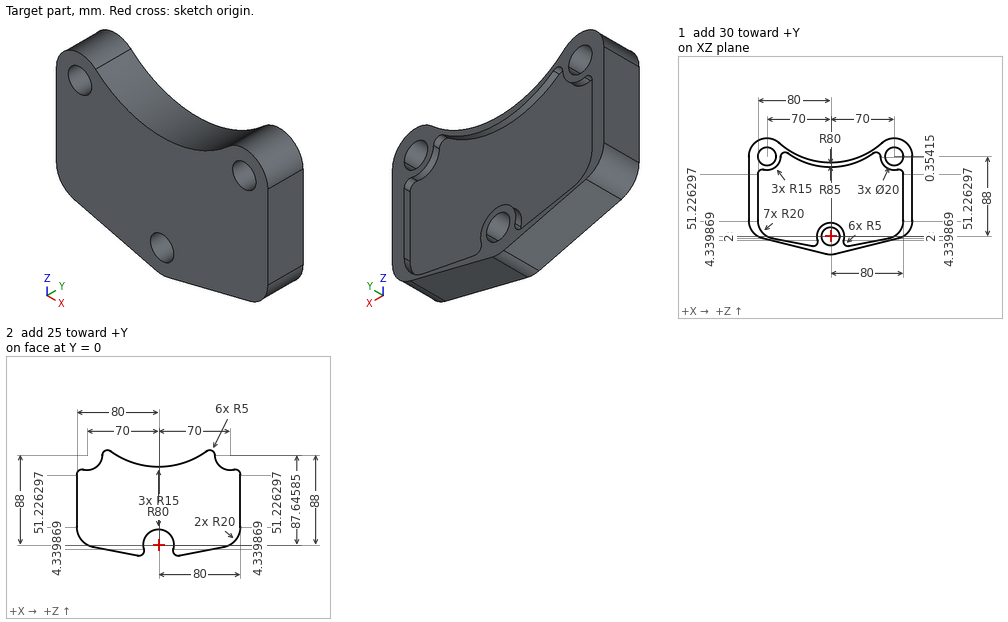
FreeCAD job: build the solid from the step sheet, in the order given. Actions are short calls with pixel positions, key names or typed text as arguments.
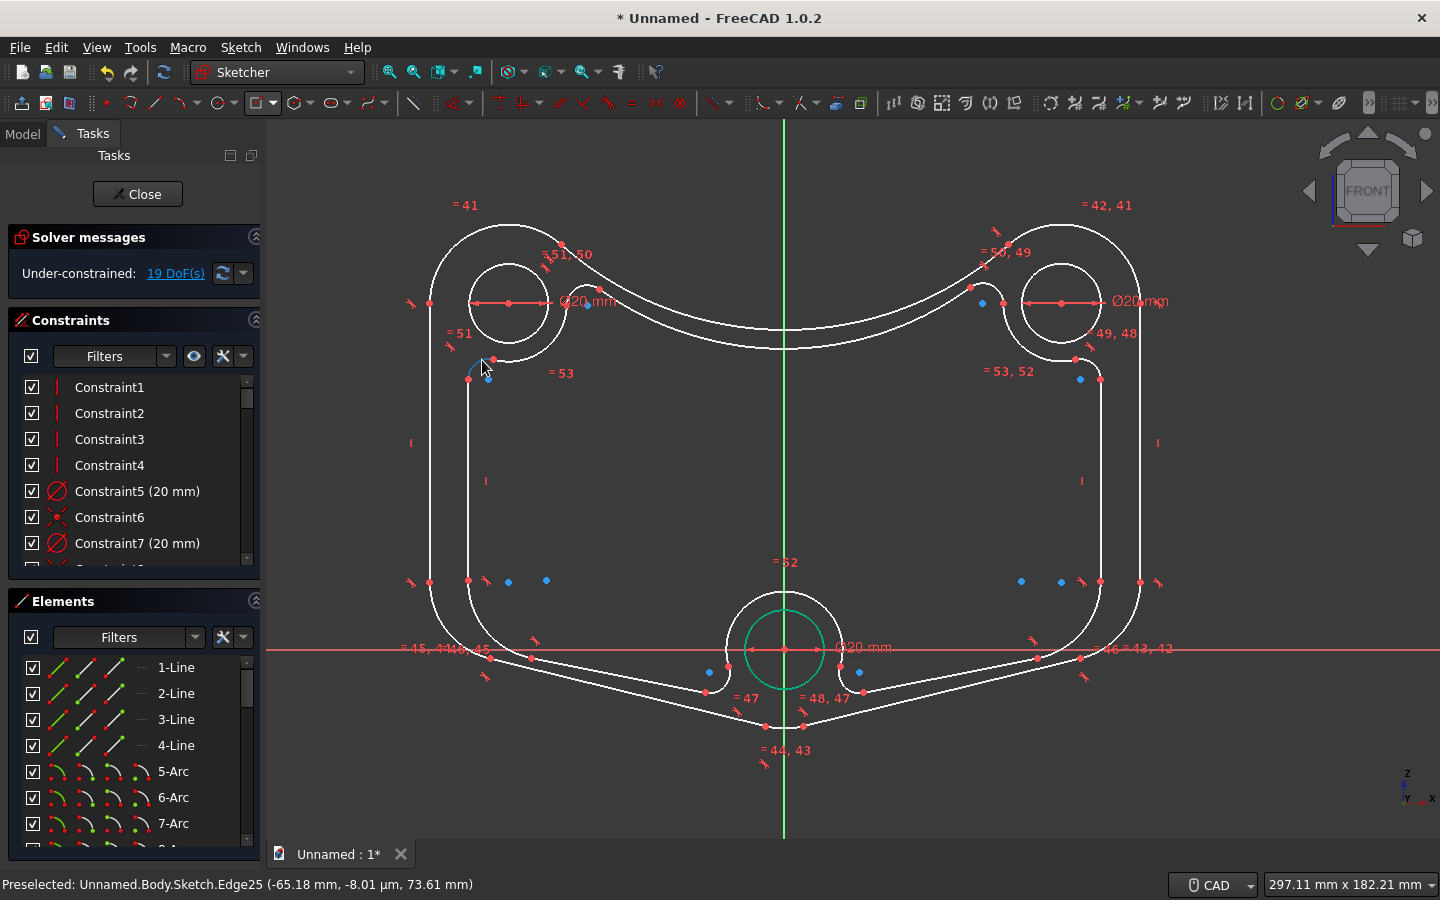
scroll(785, 719, down, 2)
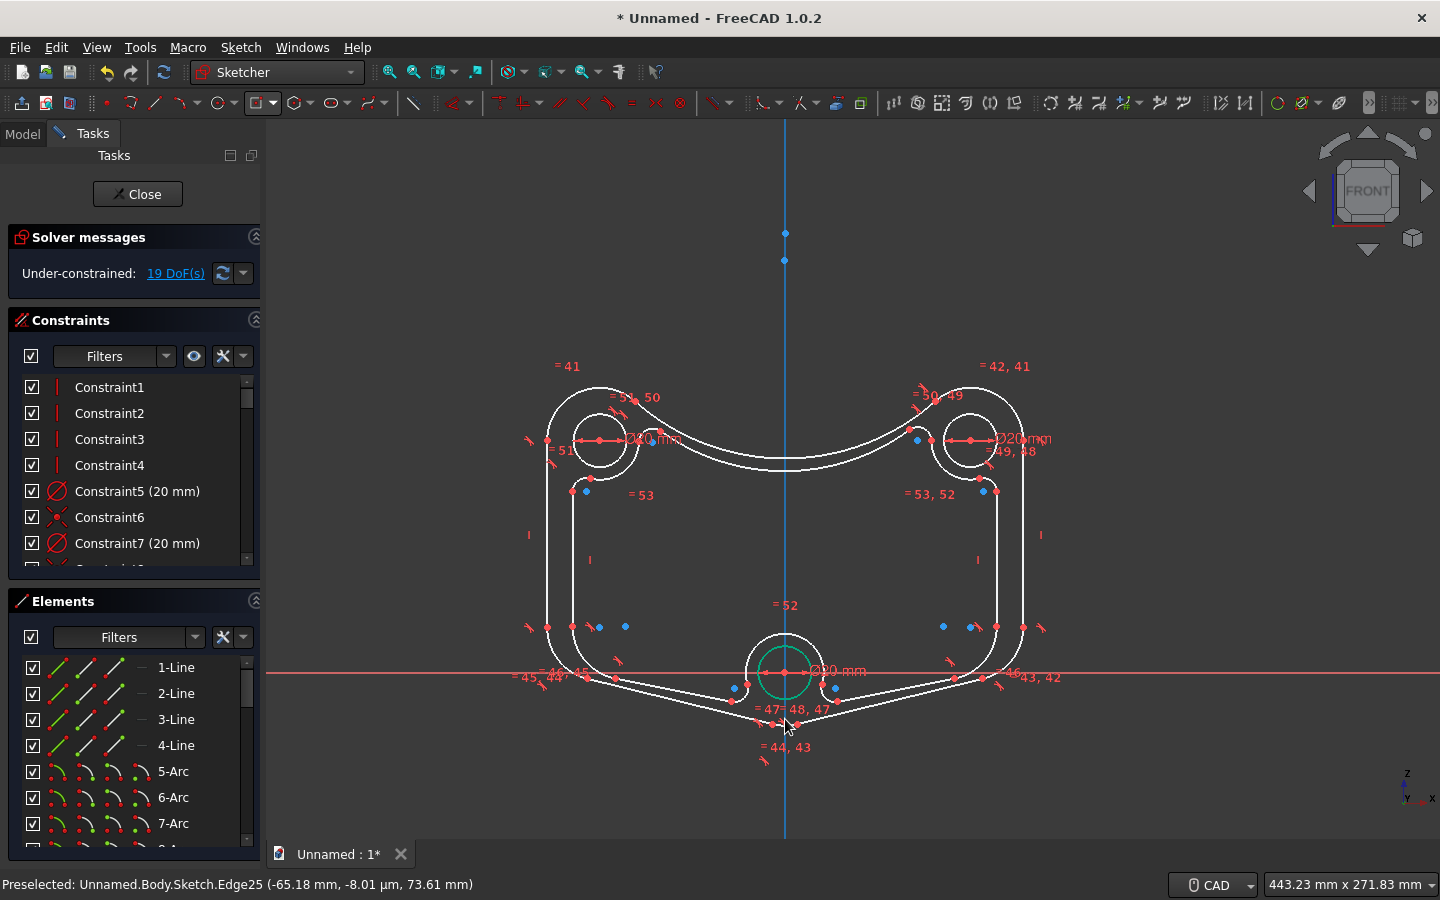
click(785, 233)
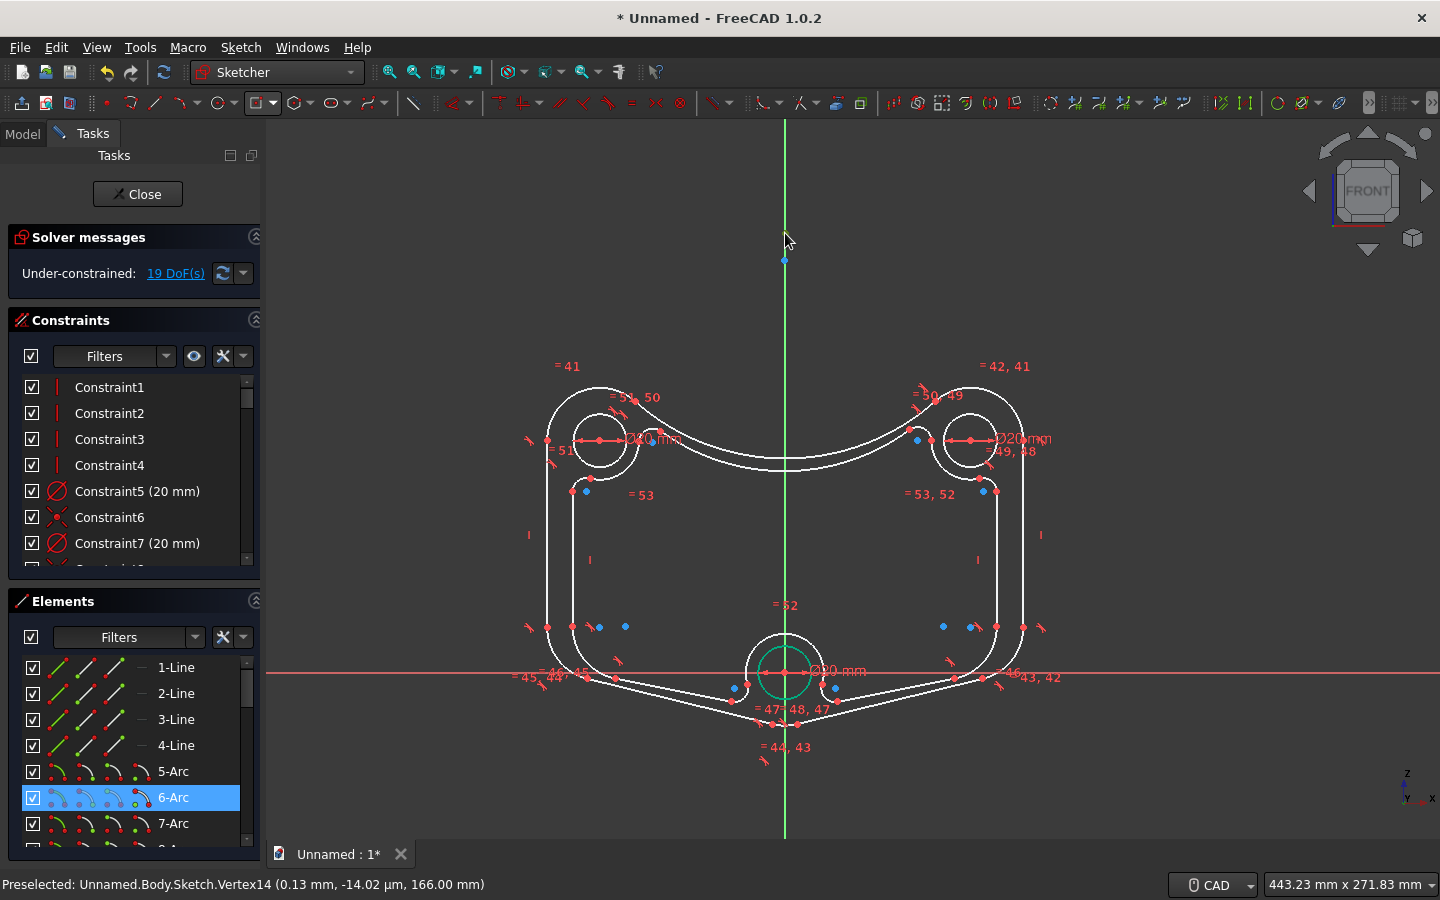
click(785, 574)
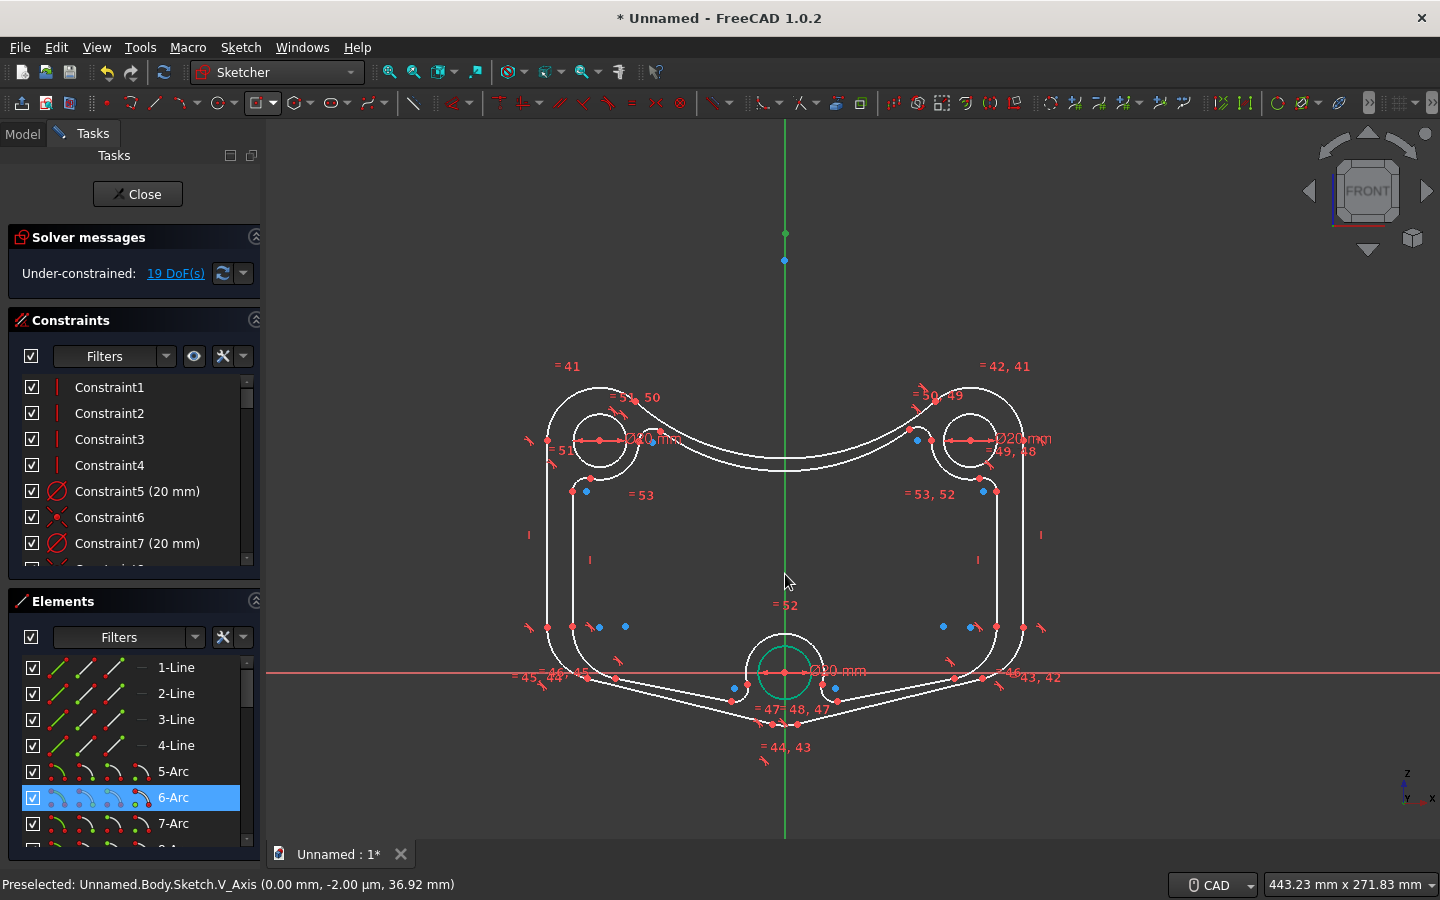
click(500, 104)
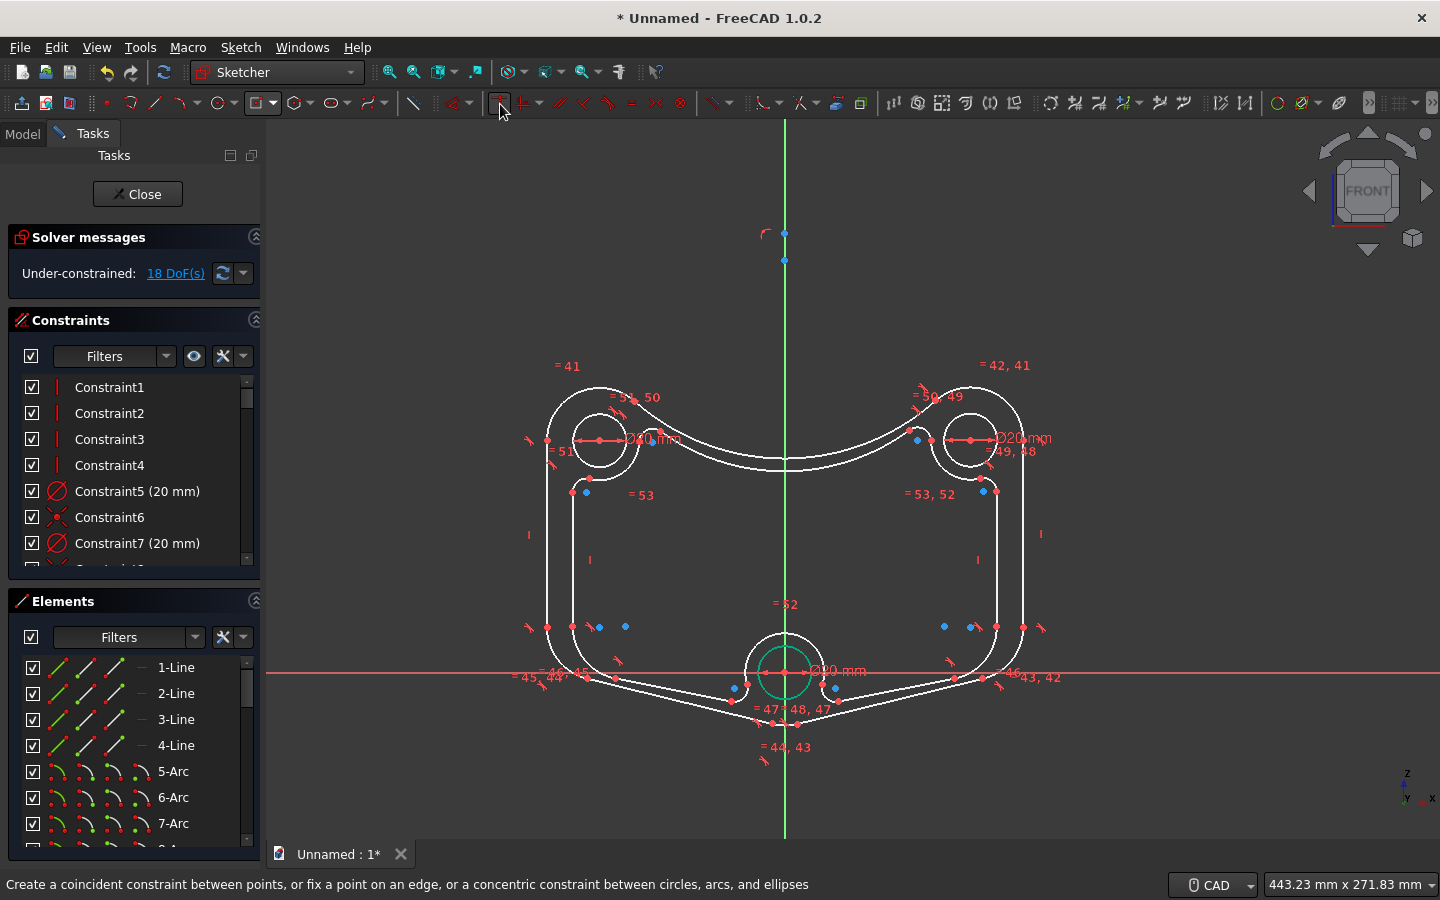
click(784, 260)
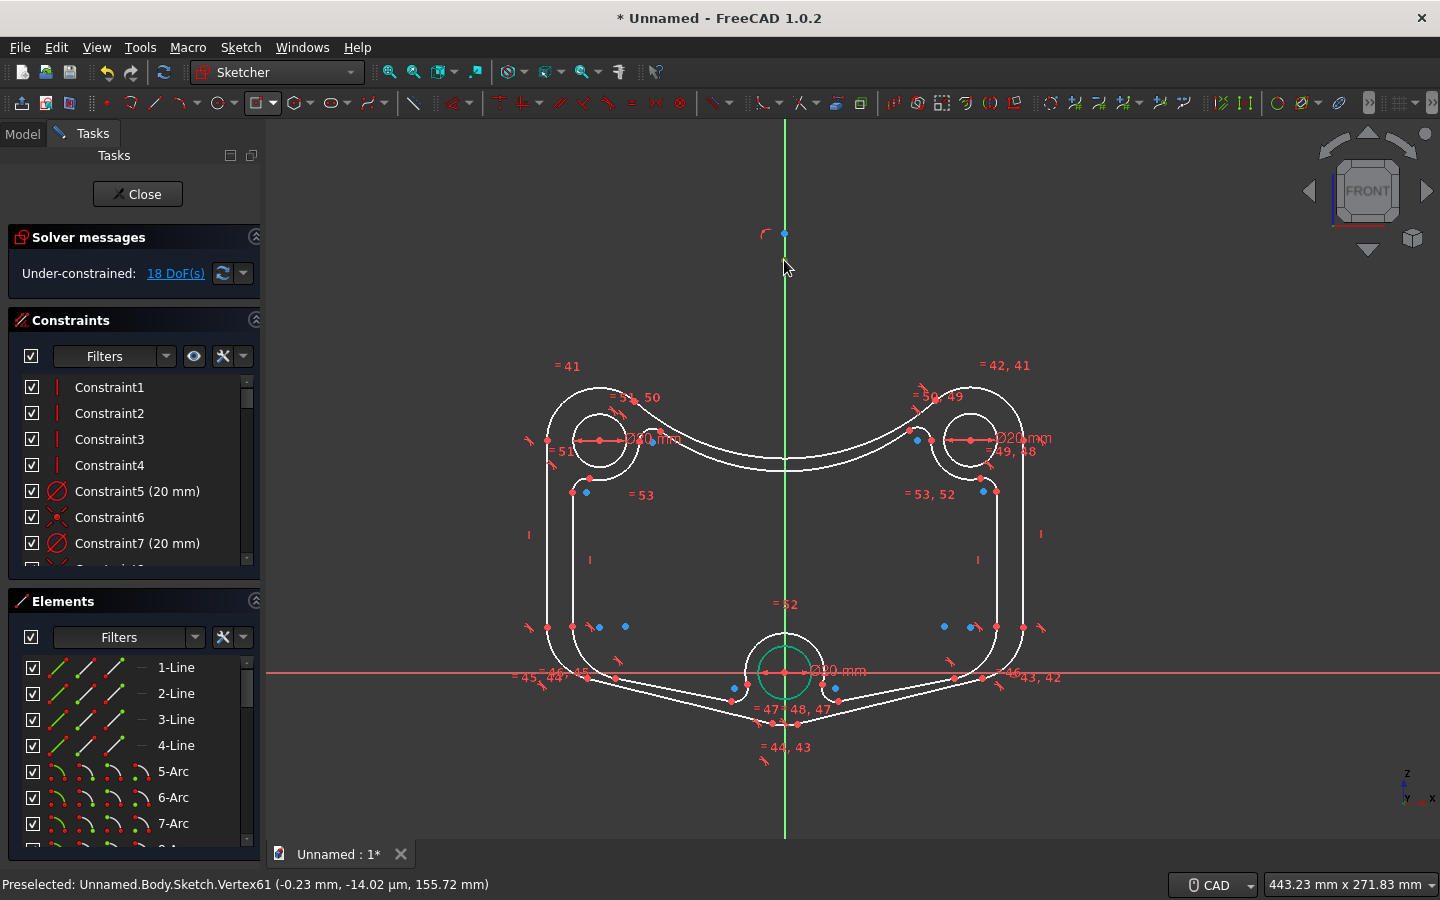
click(785, 574)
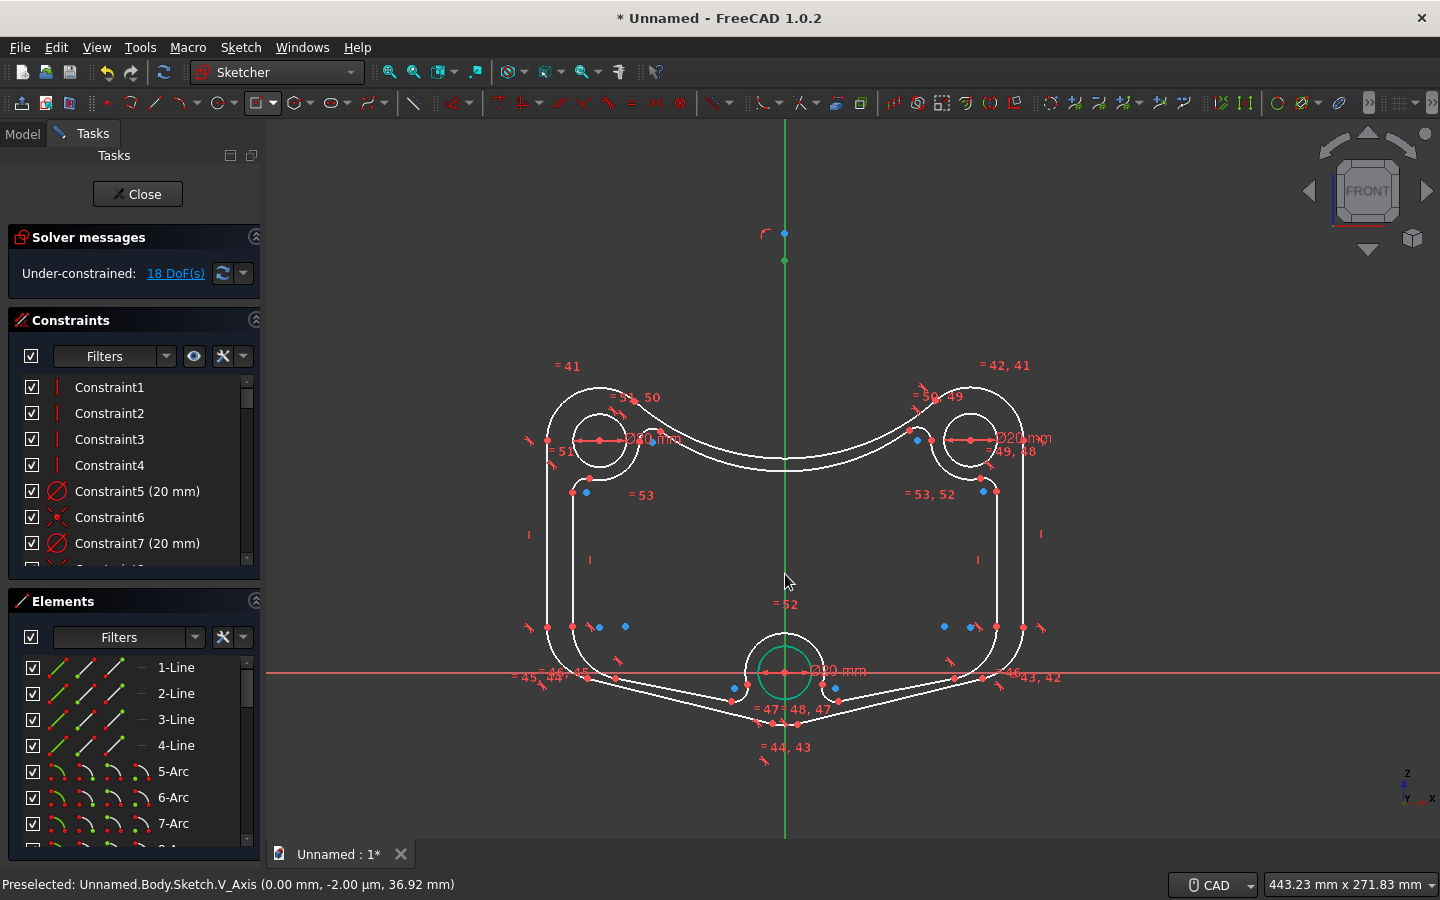
key(c)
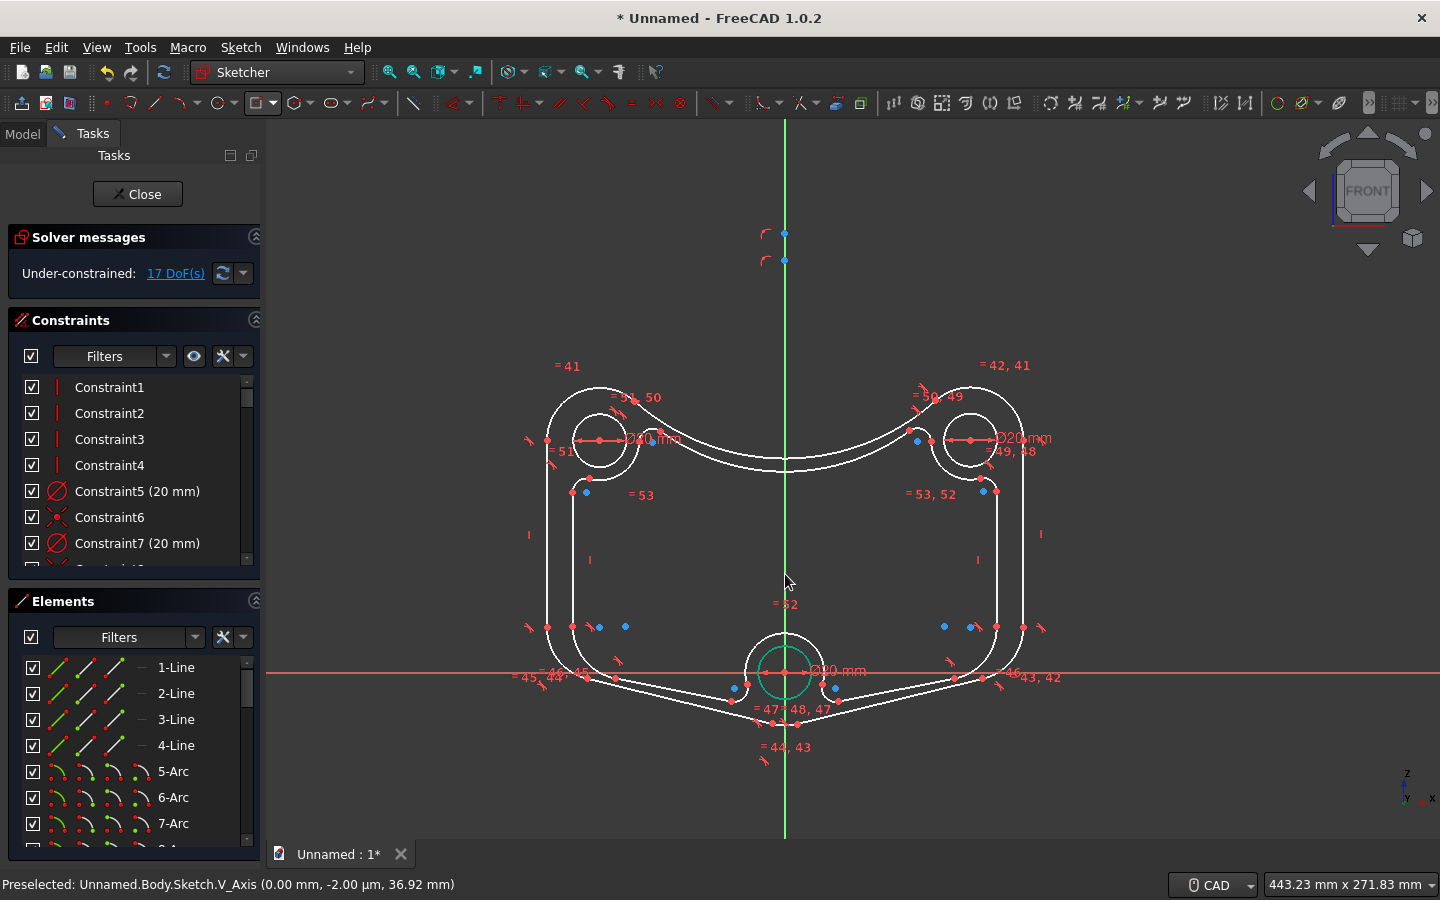
click(602, 388)